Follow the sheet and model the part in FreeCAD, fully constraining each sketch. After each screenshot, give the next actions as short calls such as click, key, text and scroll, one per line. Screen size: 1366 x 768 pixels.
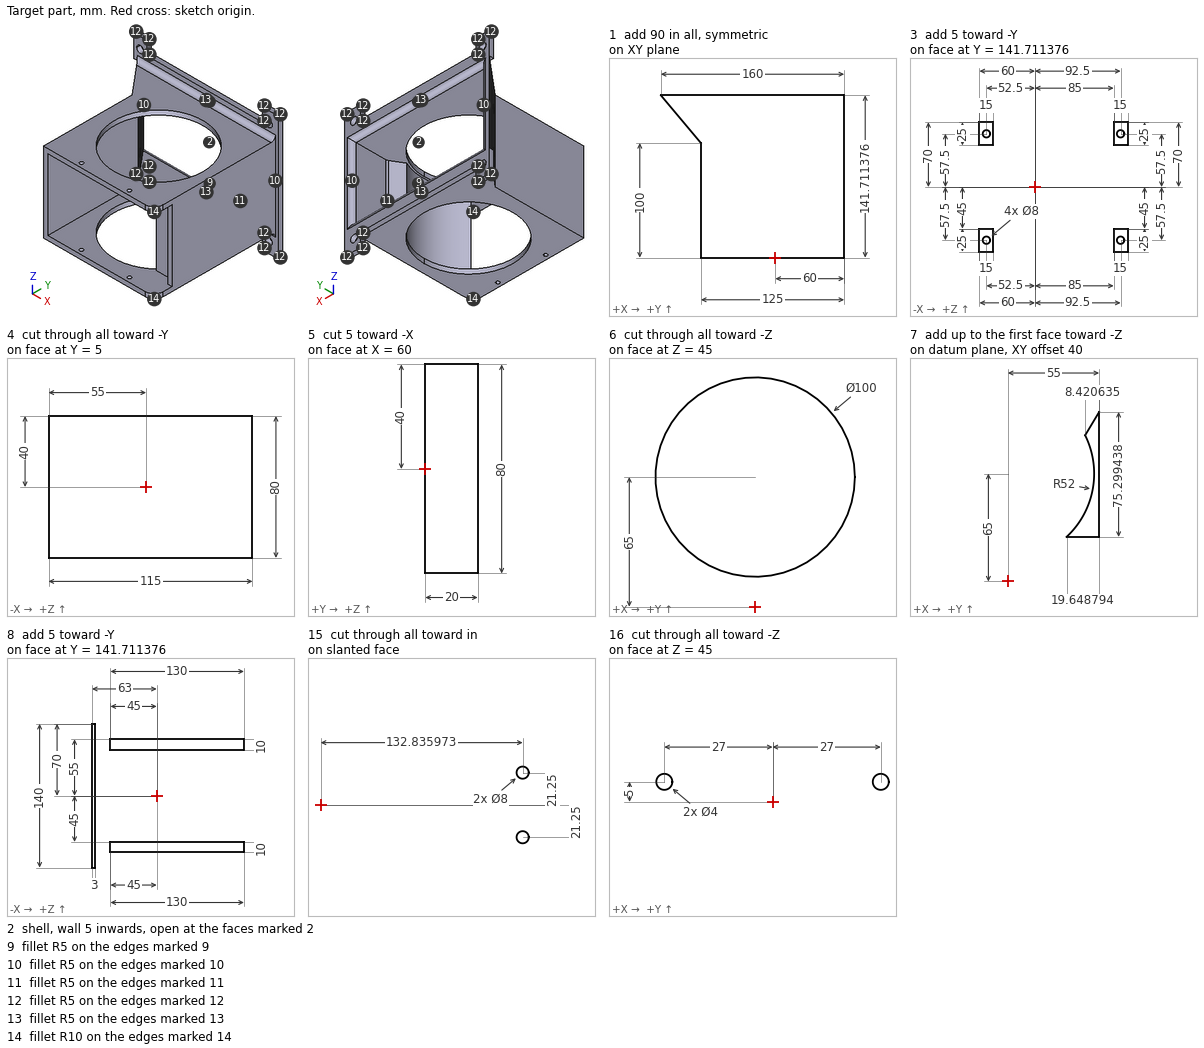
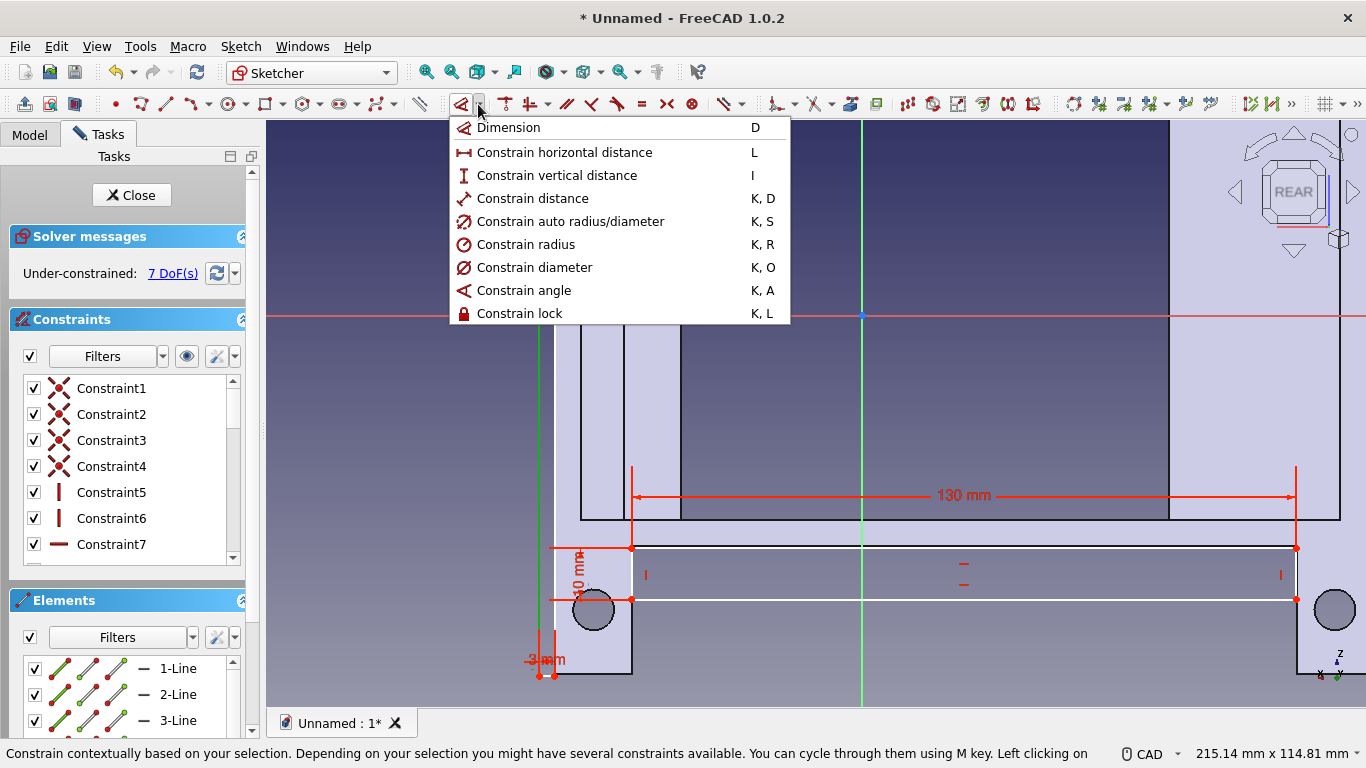
click(620, 176)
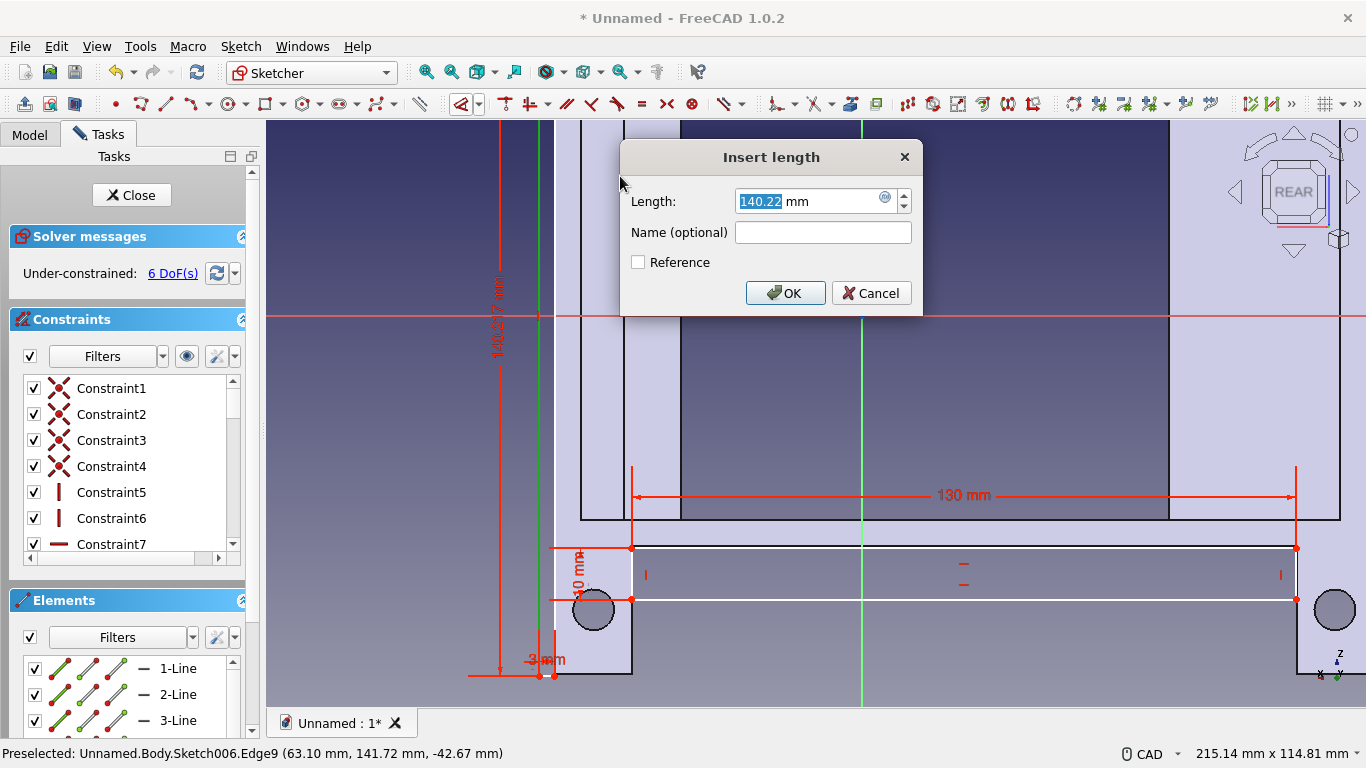
text(140)
key(Return)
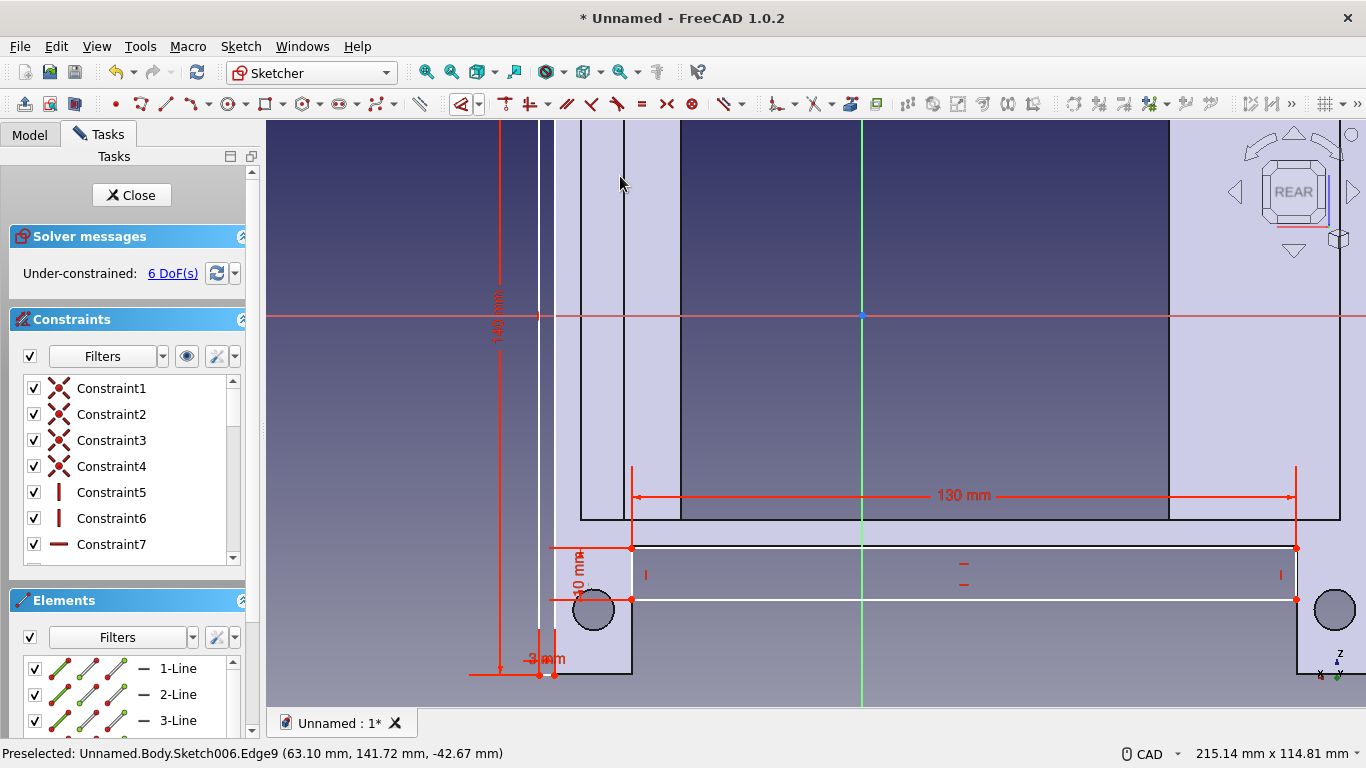
click(632, 548)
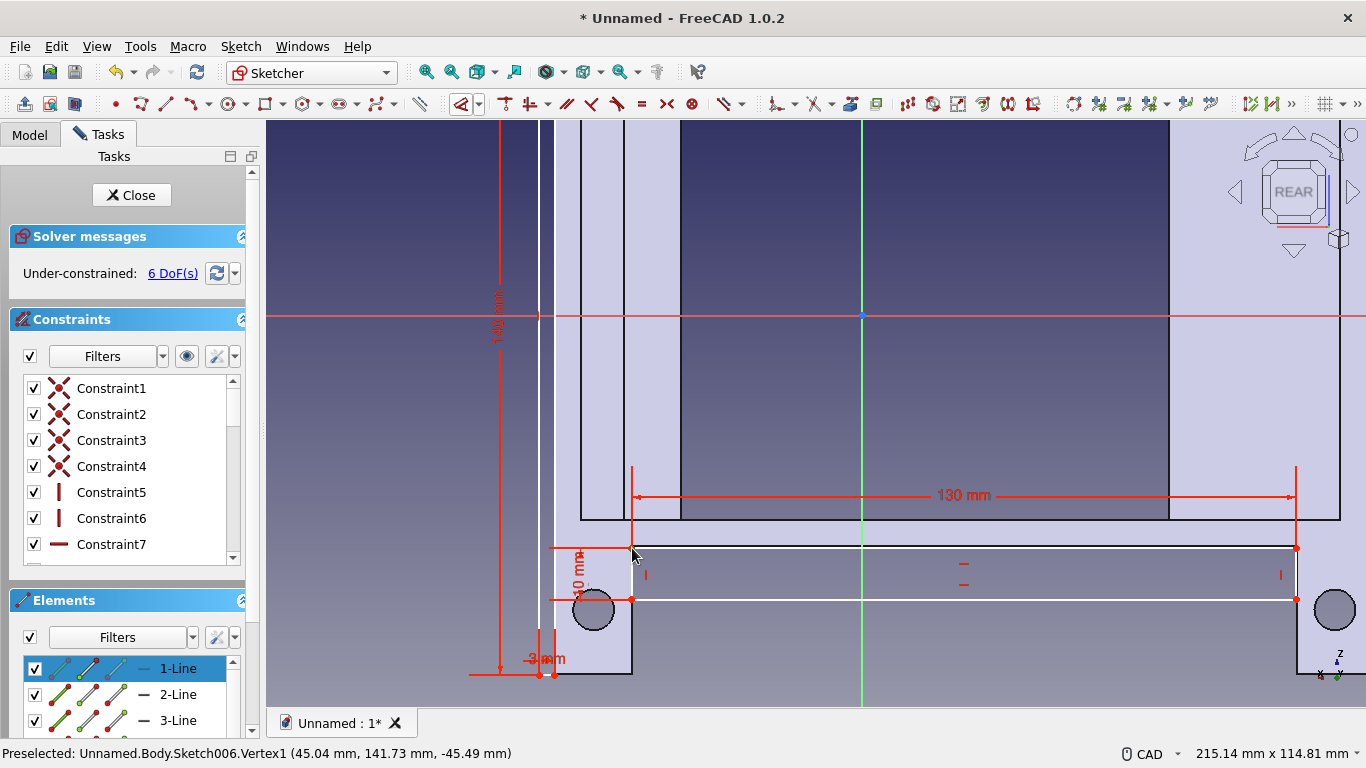
key(l)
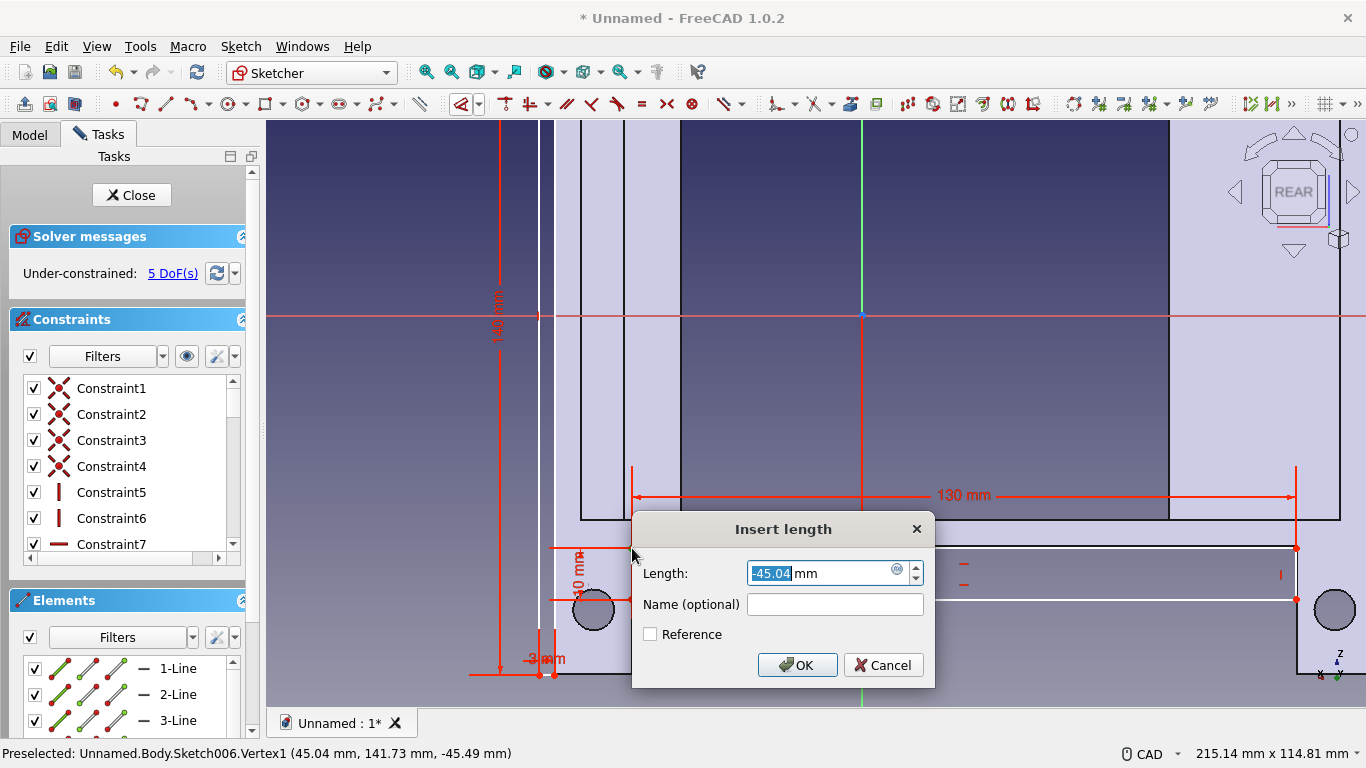
text(-45)
key(Return)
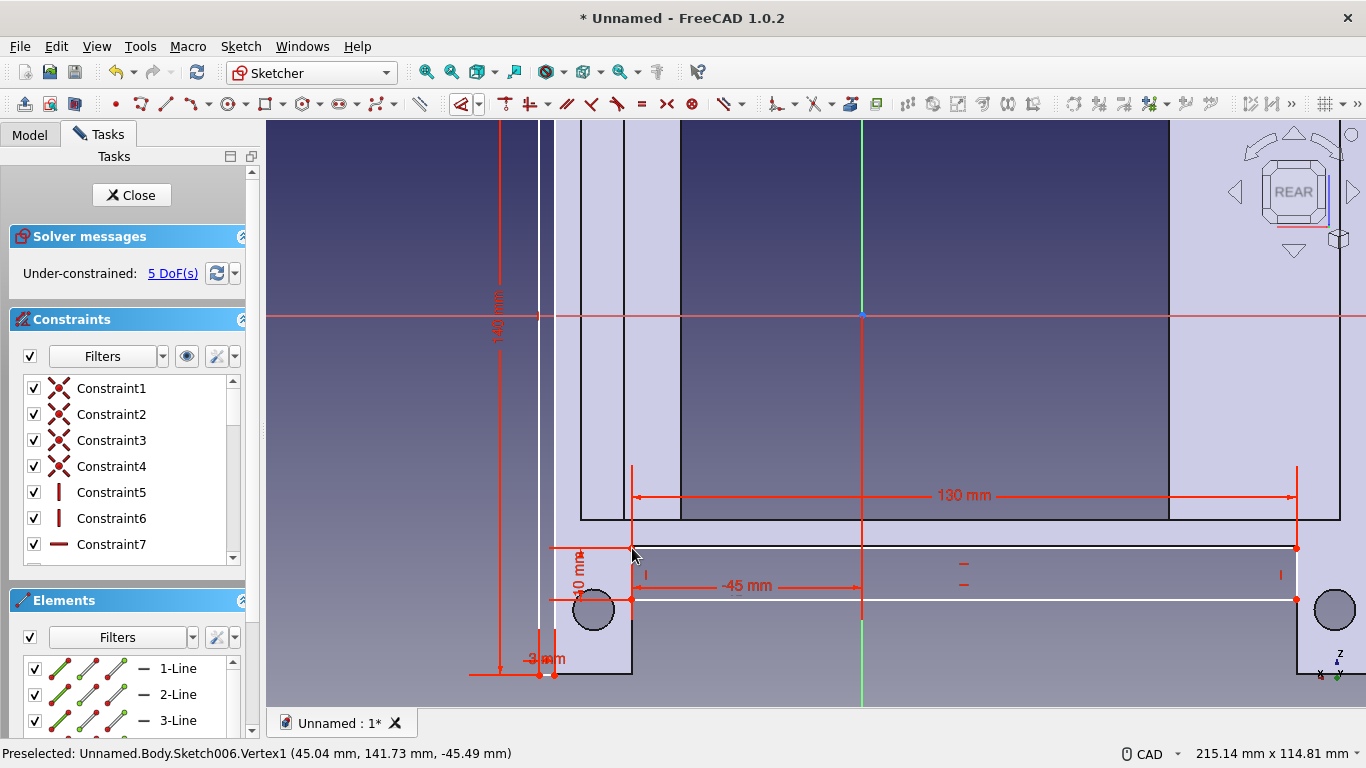
click(632, 548)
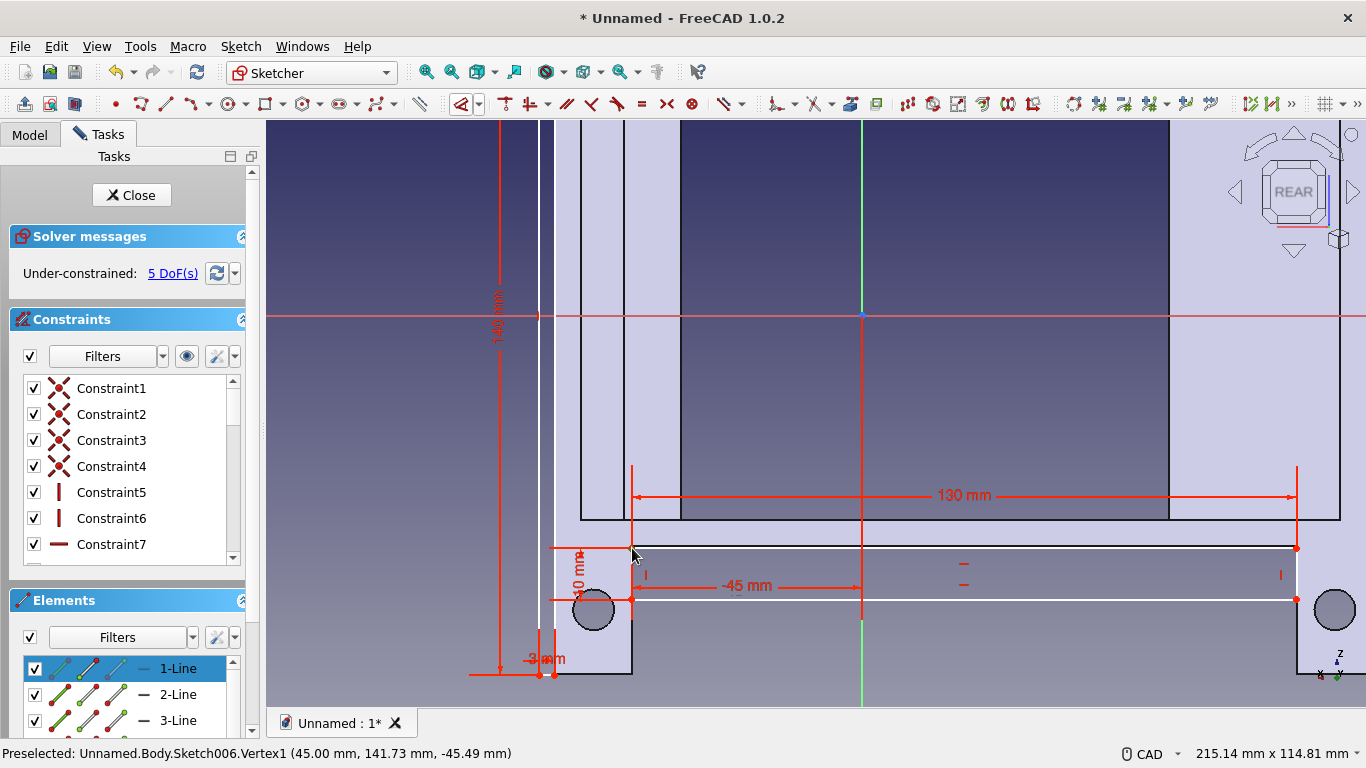
key(i)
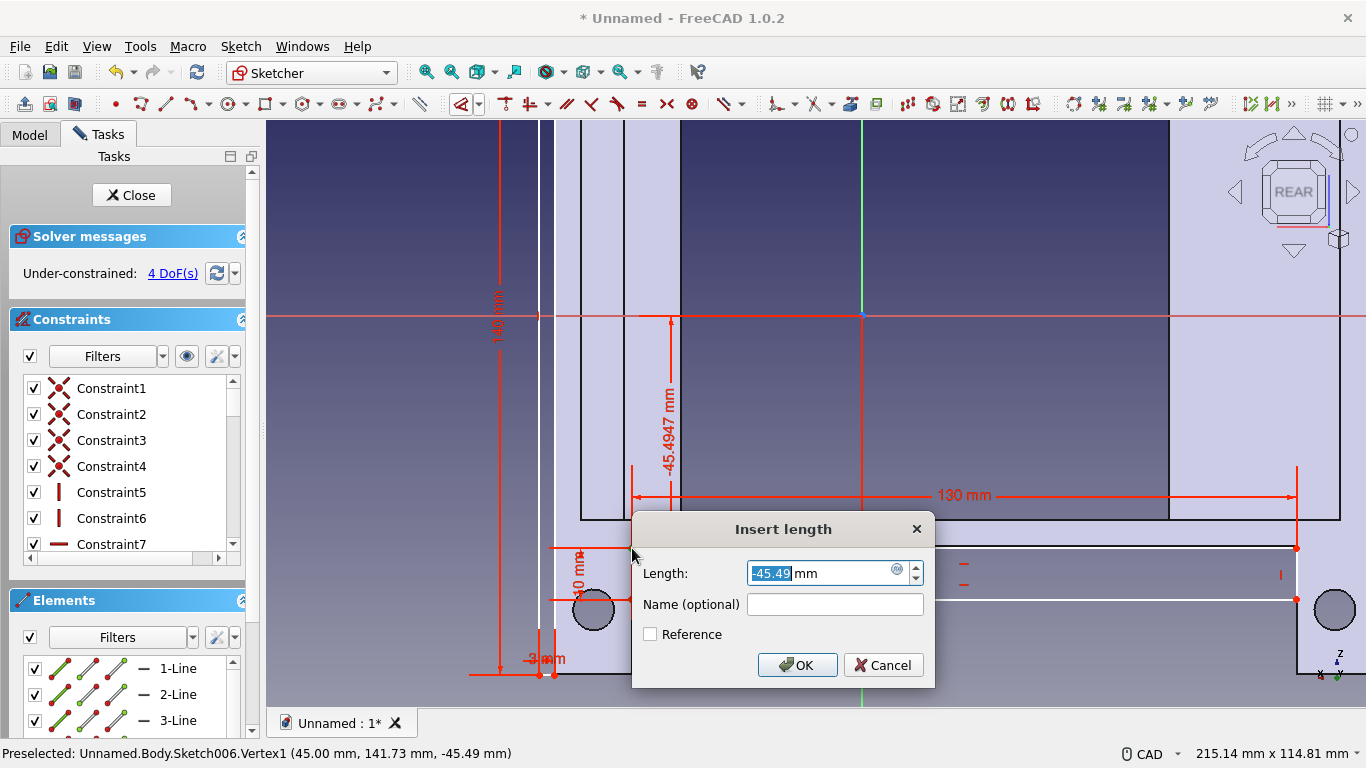
text(-45)
key(Return)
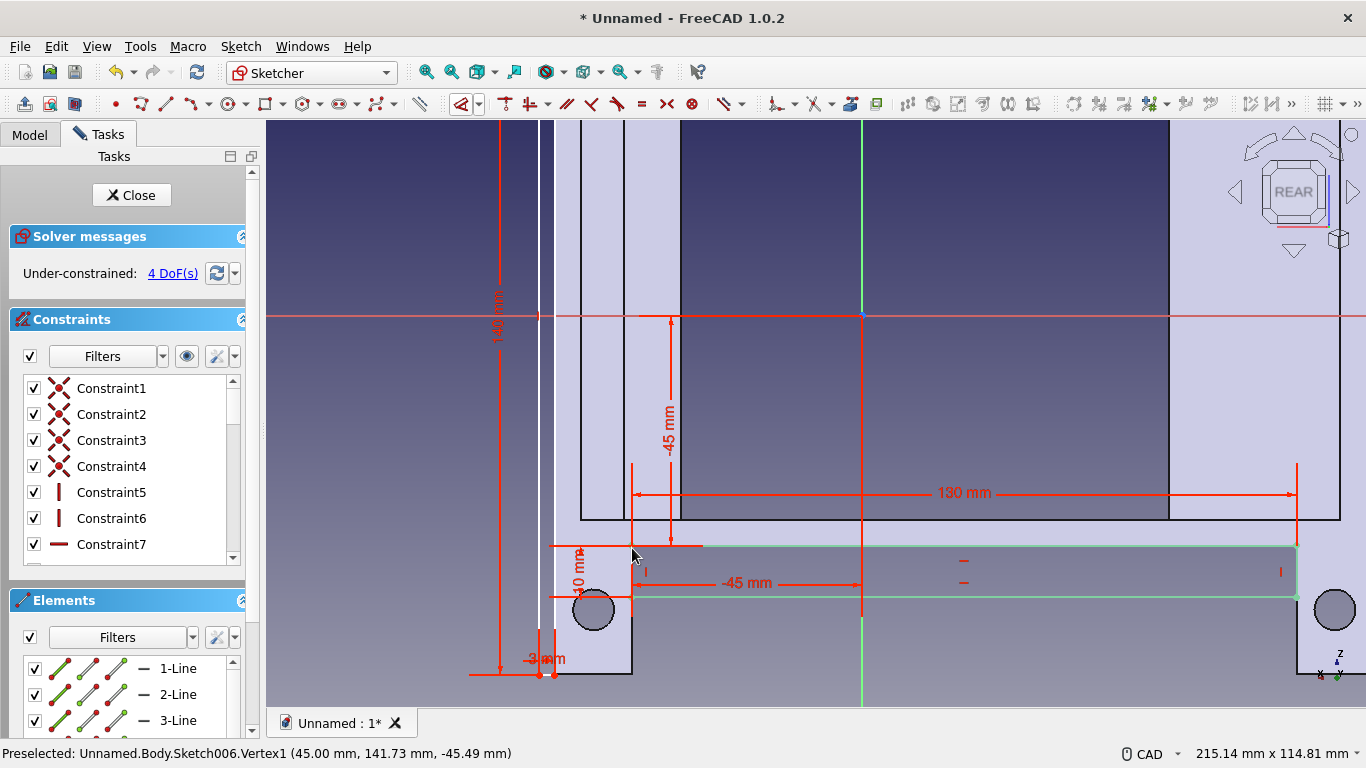
scroll(540, 532, down, 3)